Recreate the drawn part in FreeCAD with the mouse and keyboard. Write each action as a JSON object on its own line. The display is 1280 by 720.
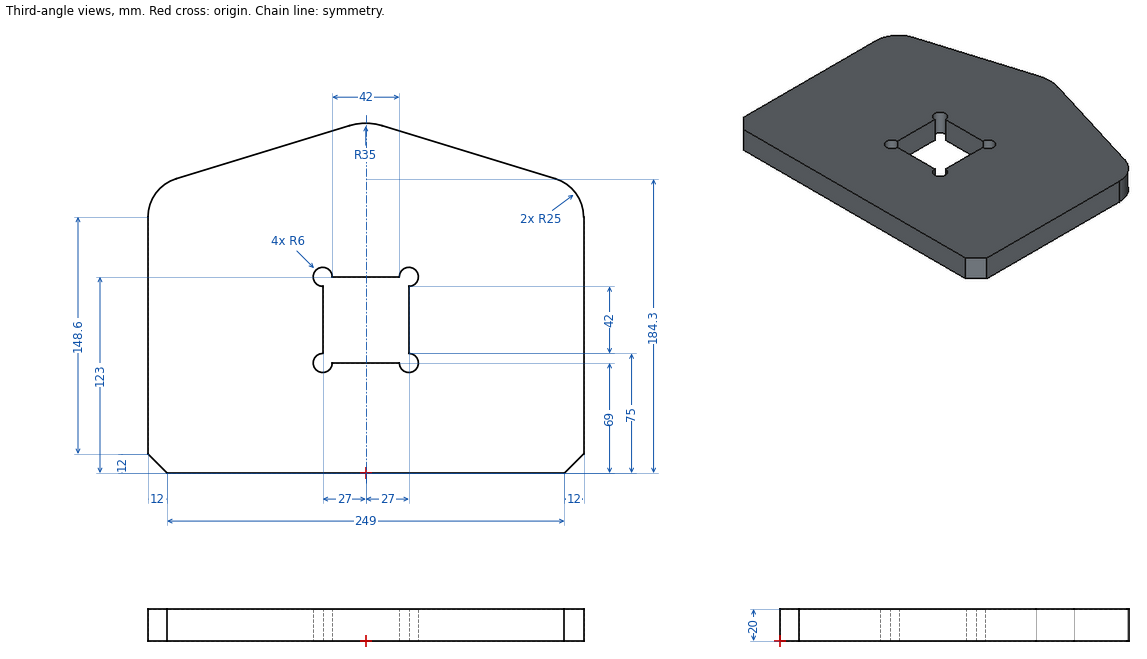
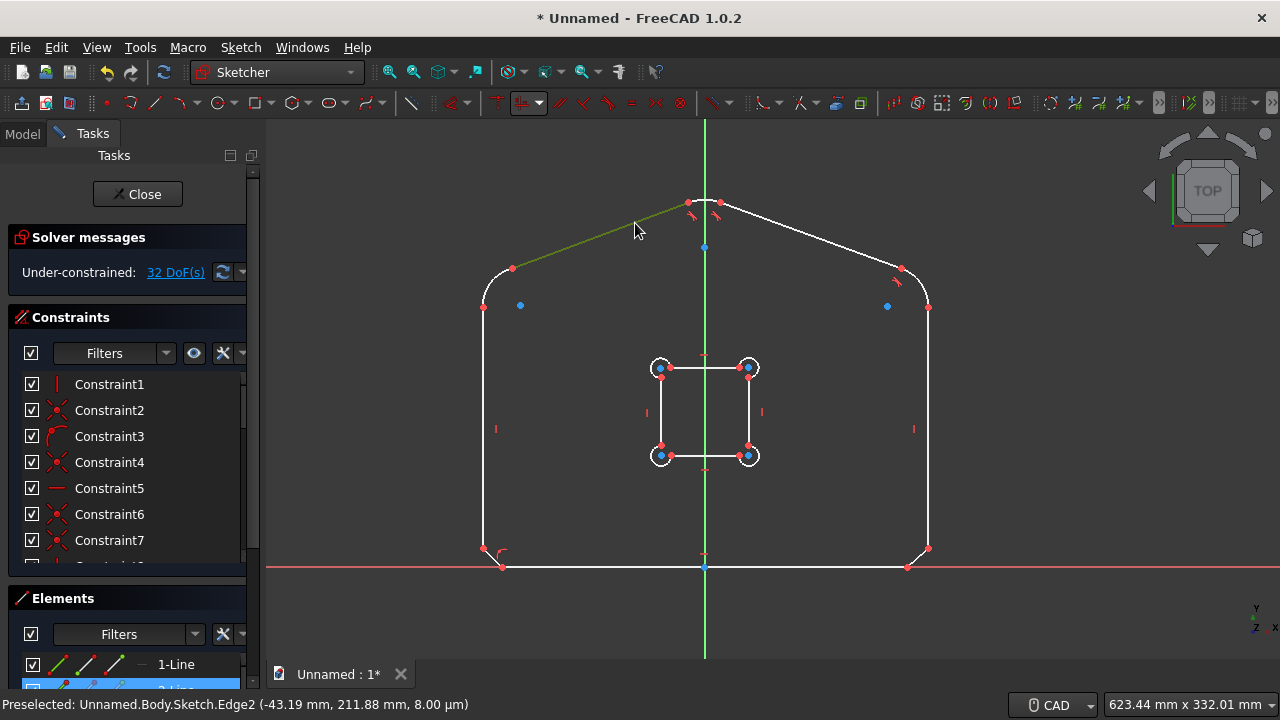
{"action": "left_click", "coordinate": [498, 275]}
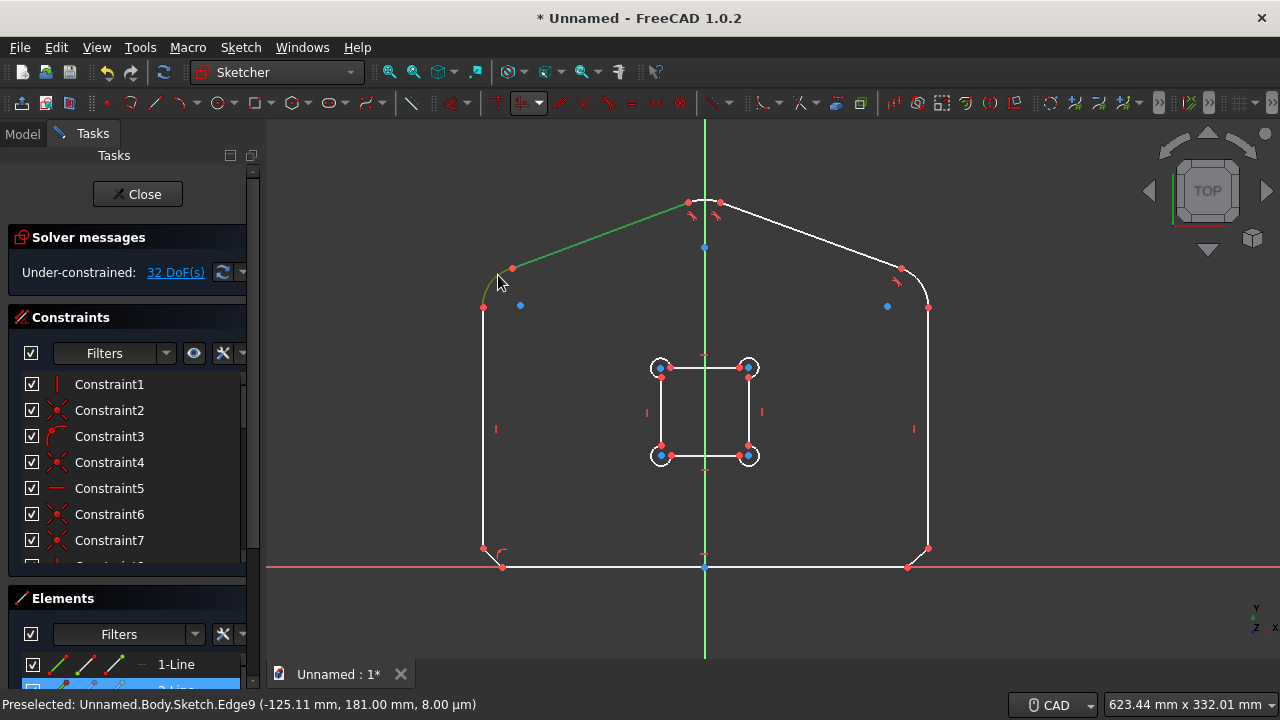
{"action": "left_click", "coordinate": [608, 104]}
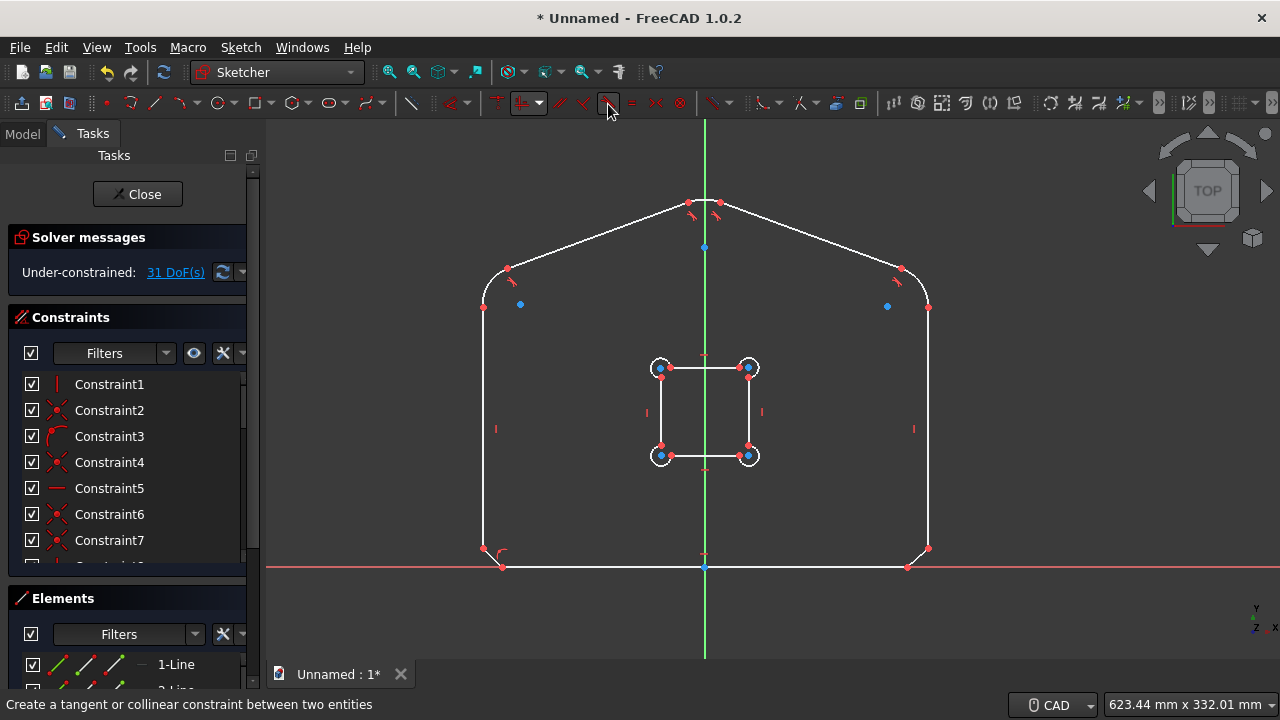
{"action": "left_click", "coordinate": [483, 380]}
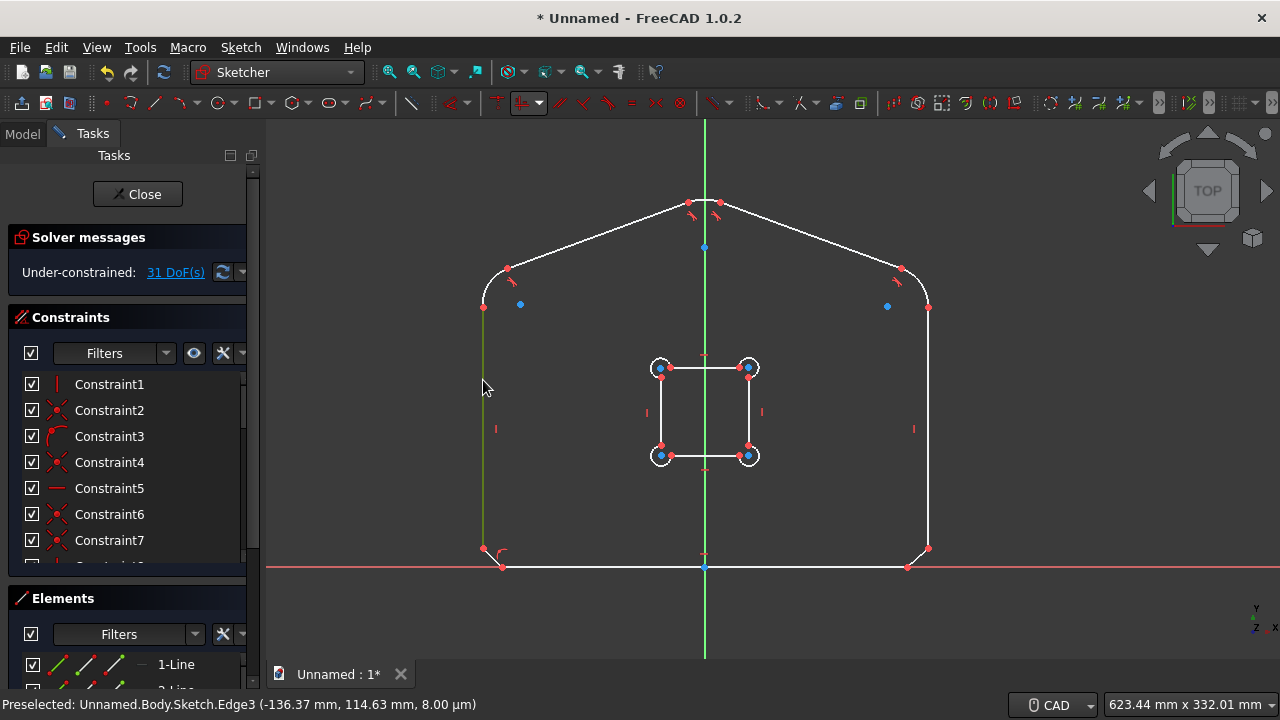
{"action": "left_click", "coordinate": [495, 276]}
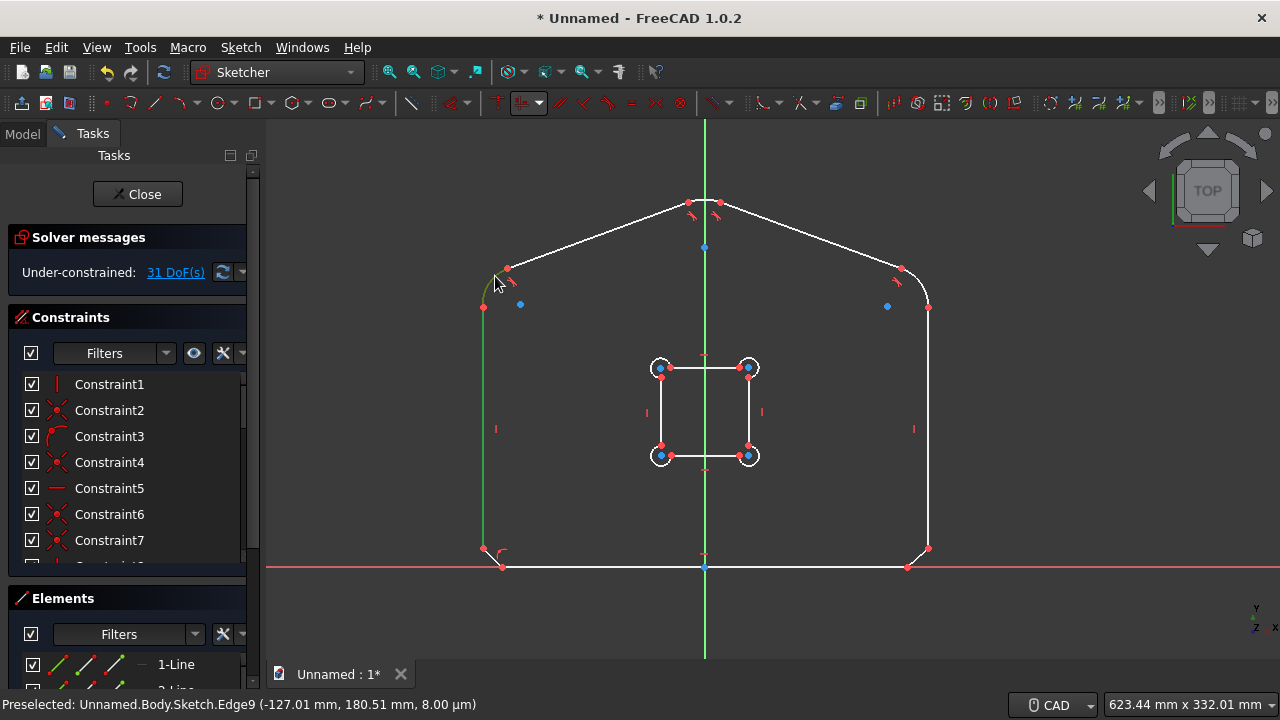
{"action": "left_click", "coordinate": [608, 104]}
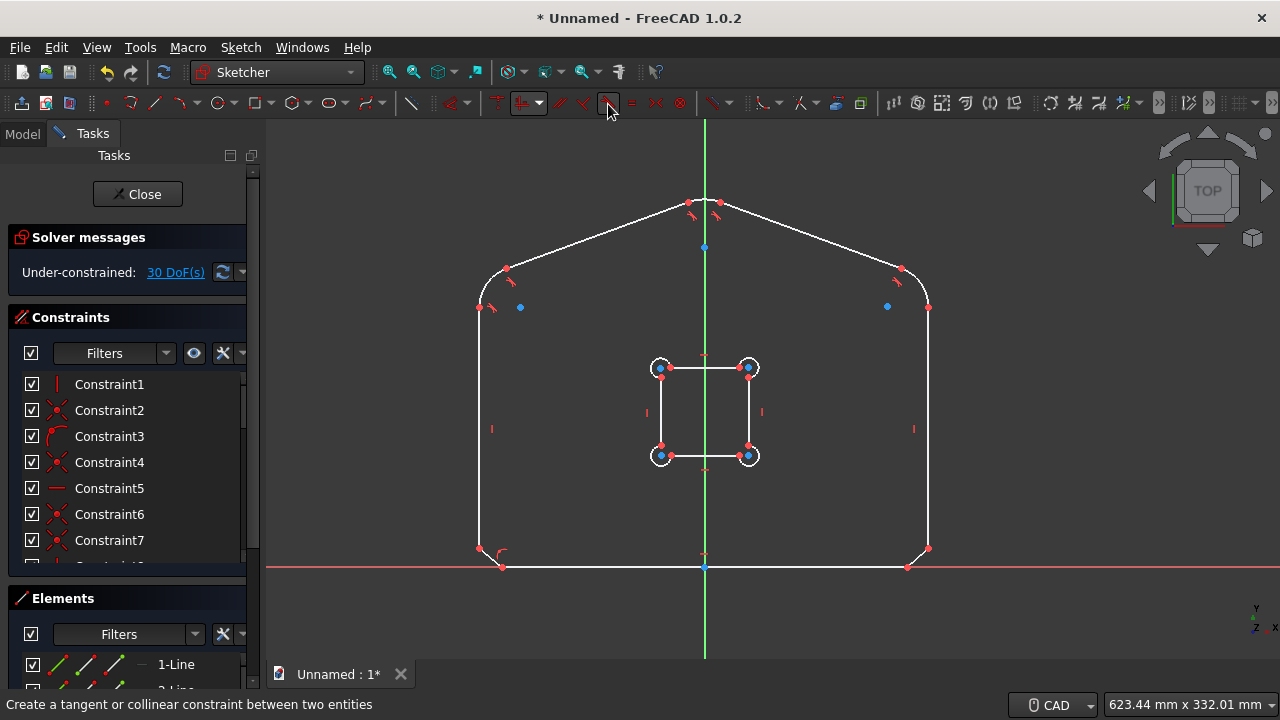
{"action": "left_click", "coordinate": [928, 476]}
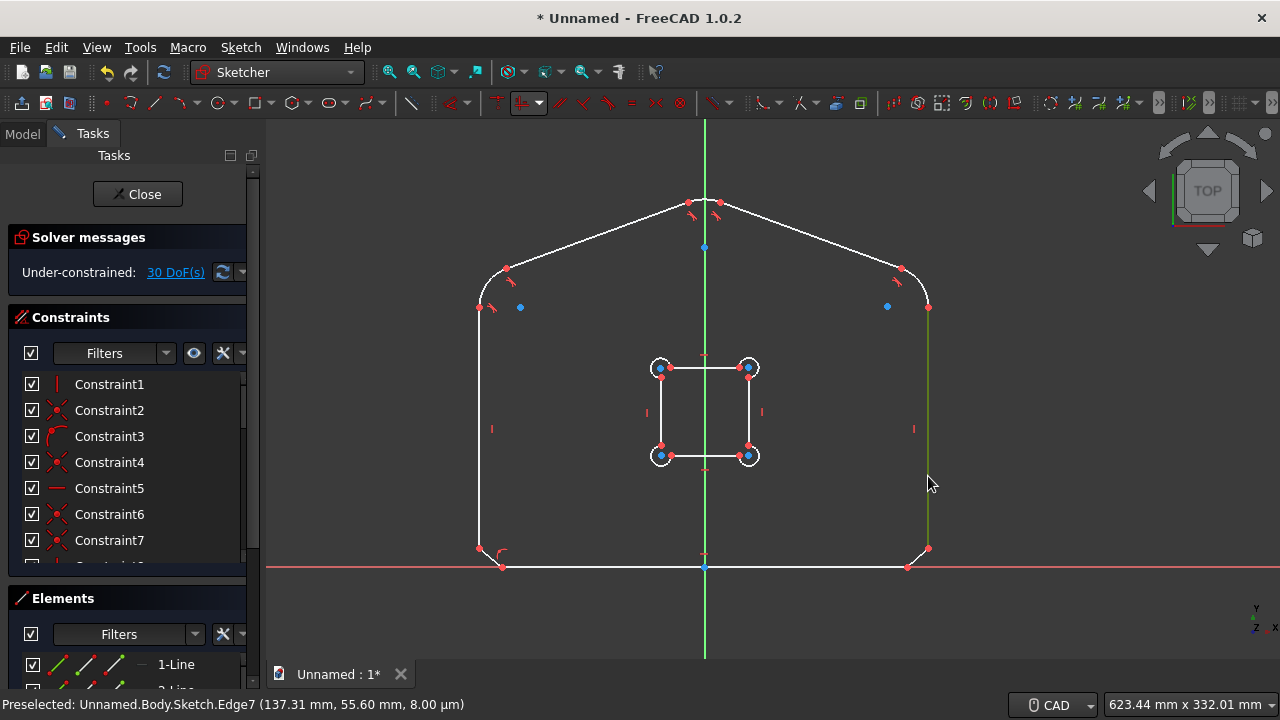
{"action": "left_click", "coordinate": [926, 293]}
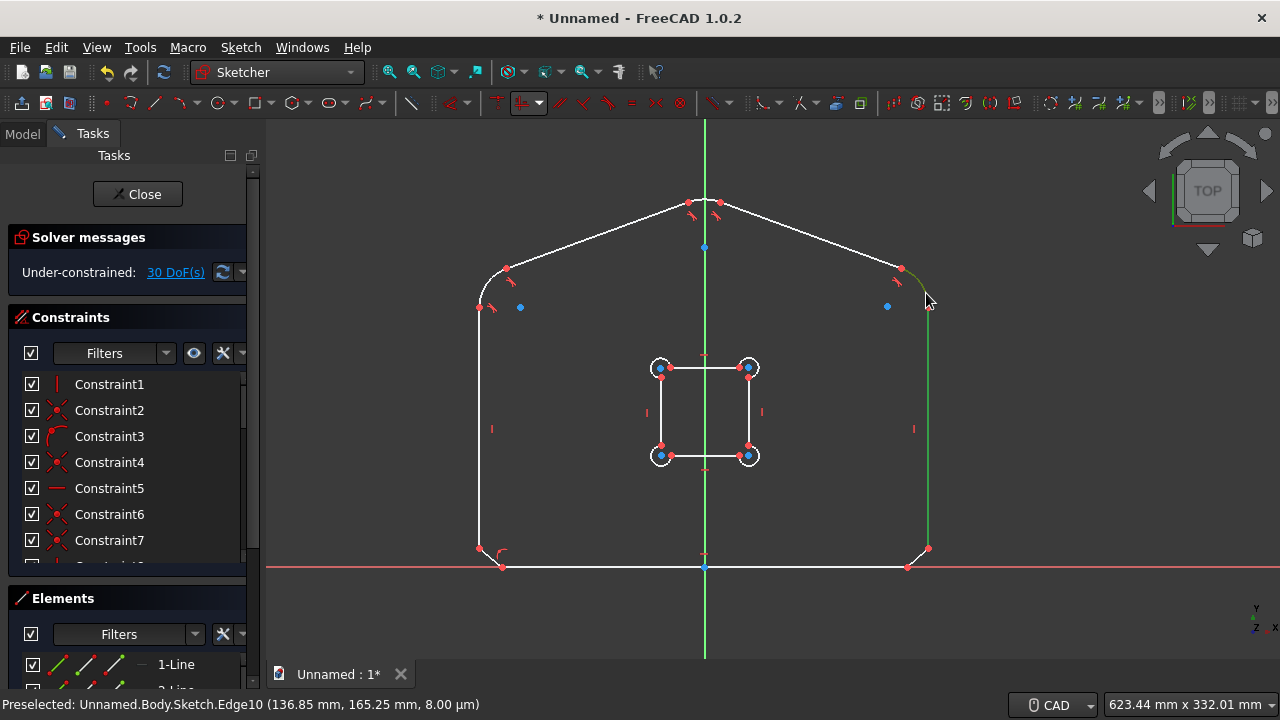
{"action": "left_click", "coordinate": [608, 104]}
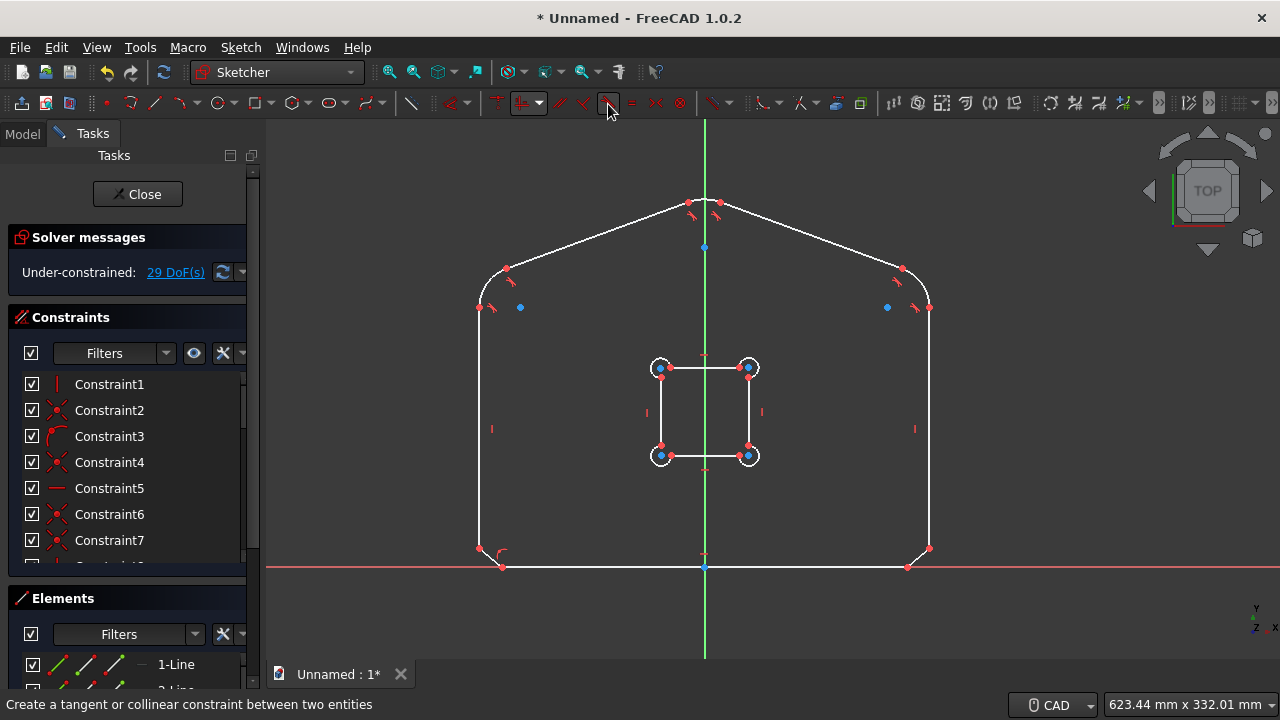
{"action": "left_click", "coordinate": [494, 276]}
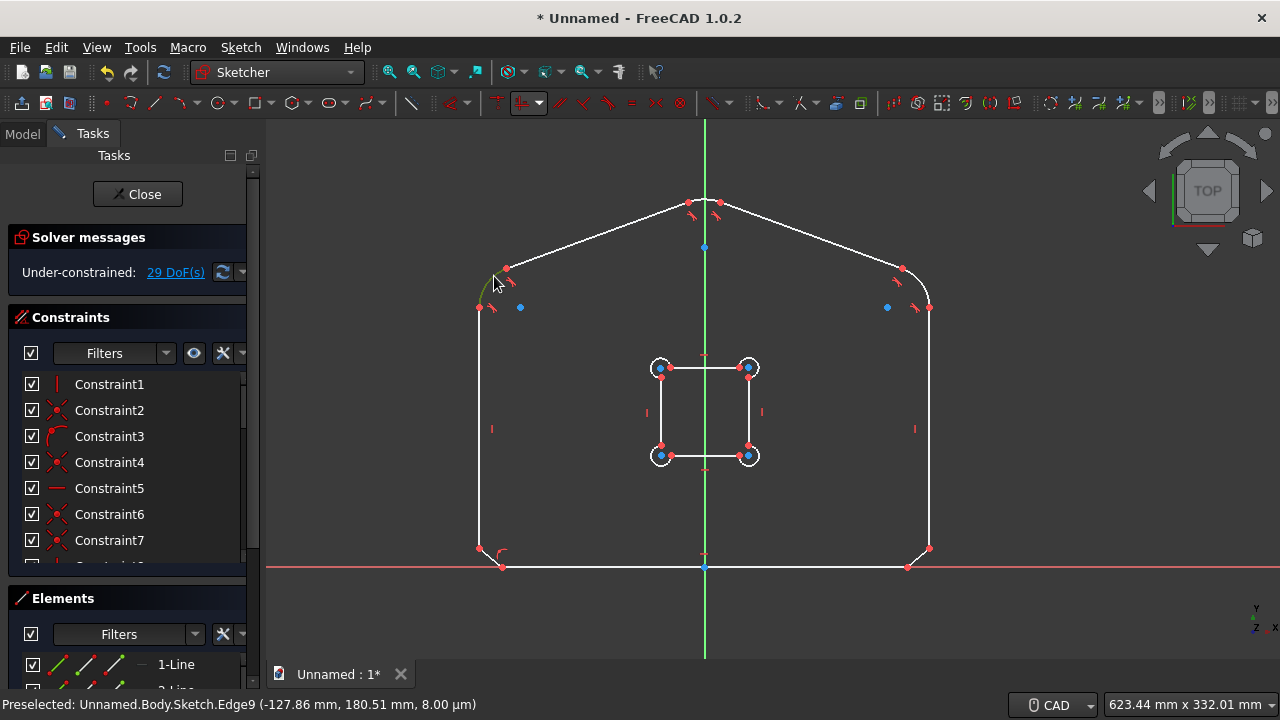
{"action": "left_click", "coordinate": [927, 293]}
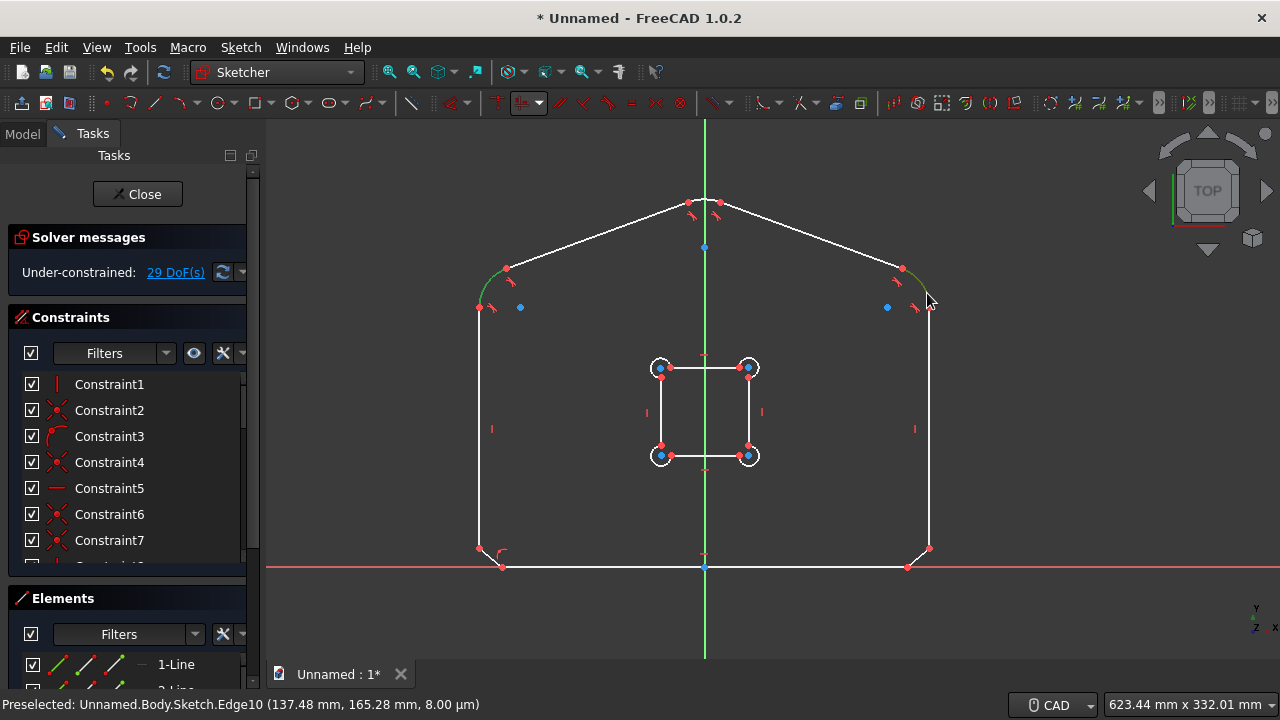
{"action": "left_click", "coordinate": [632, 104]}